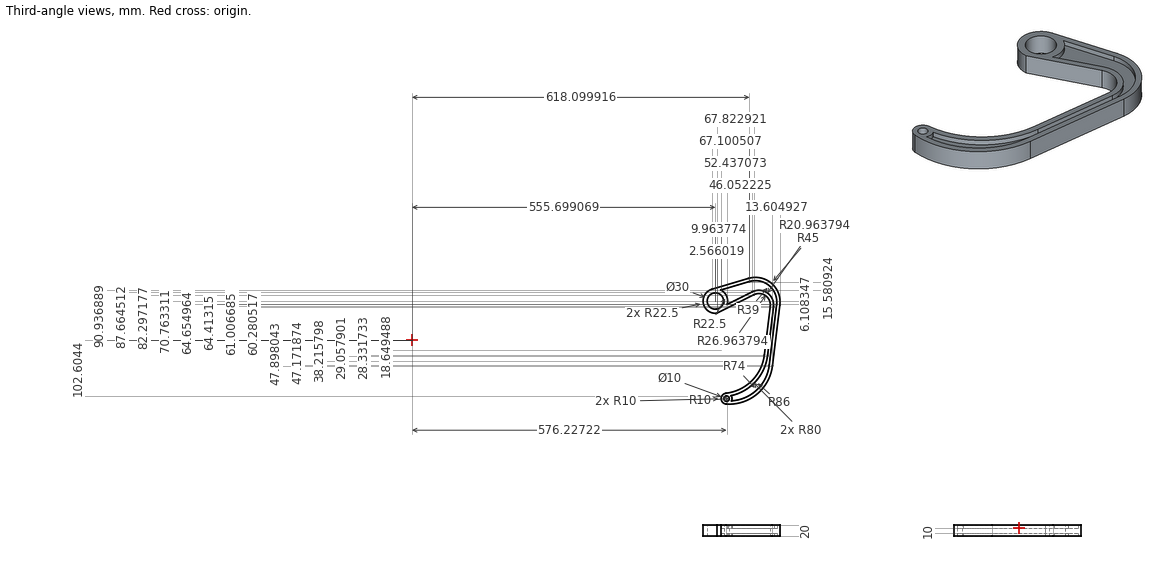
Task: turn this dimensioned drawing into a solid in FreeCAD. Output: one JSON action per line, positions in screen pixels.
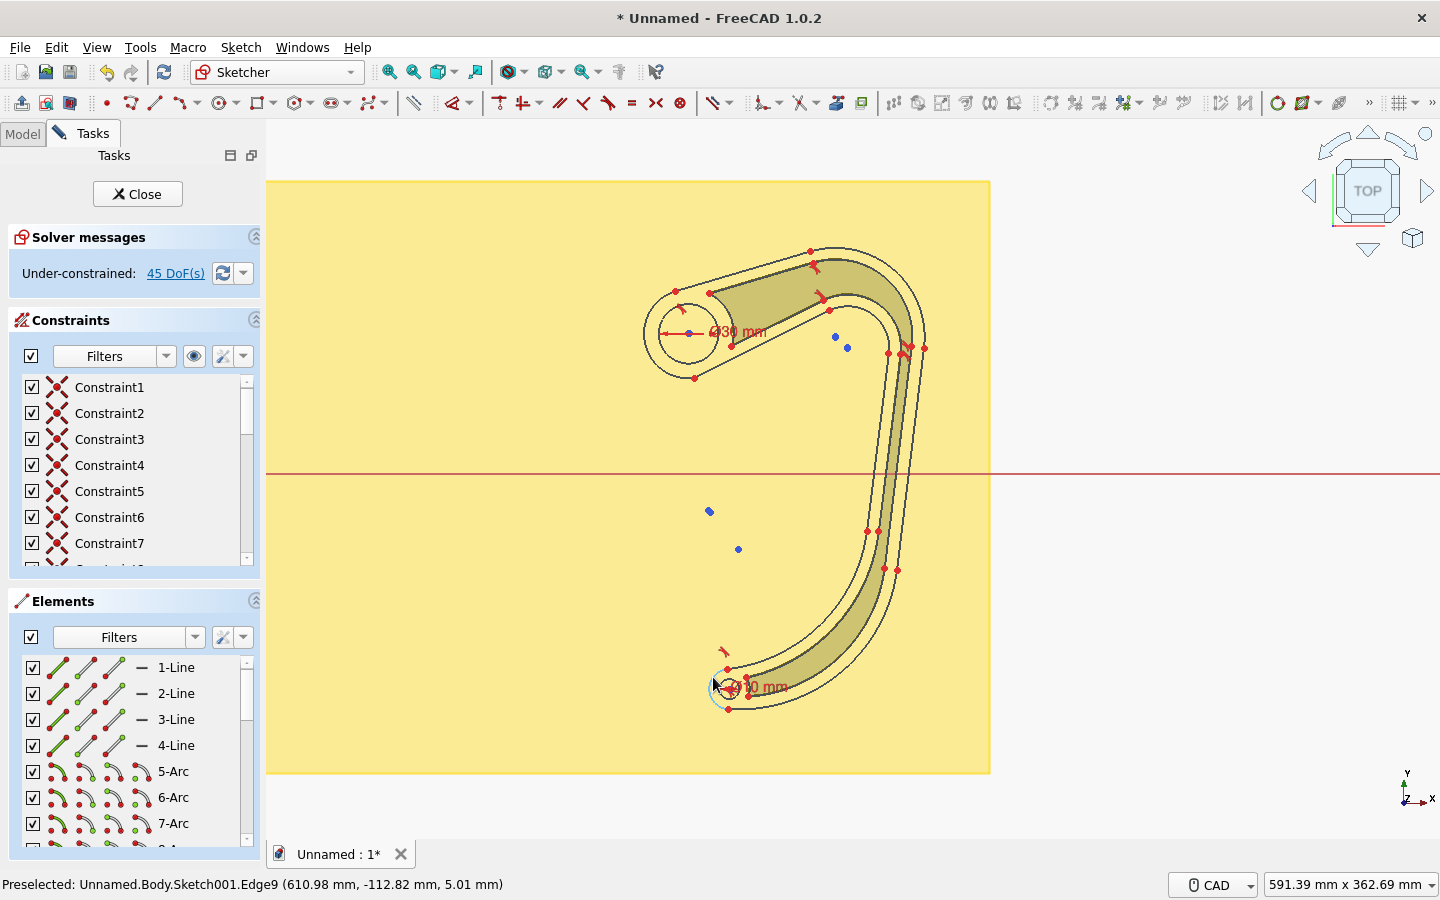
{"action": "left_click", "coordinate": [740, 285]}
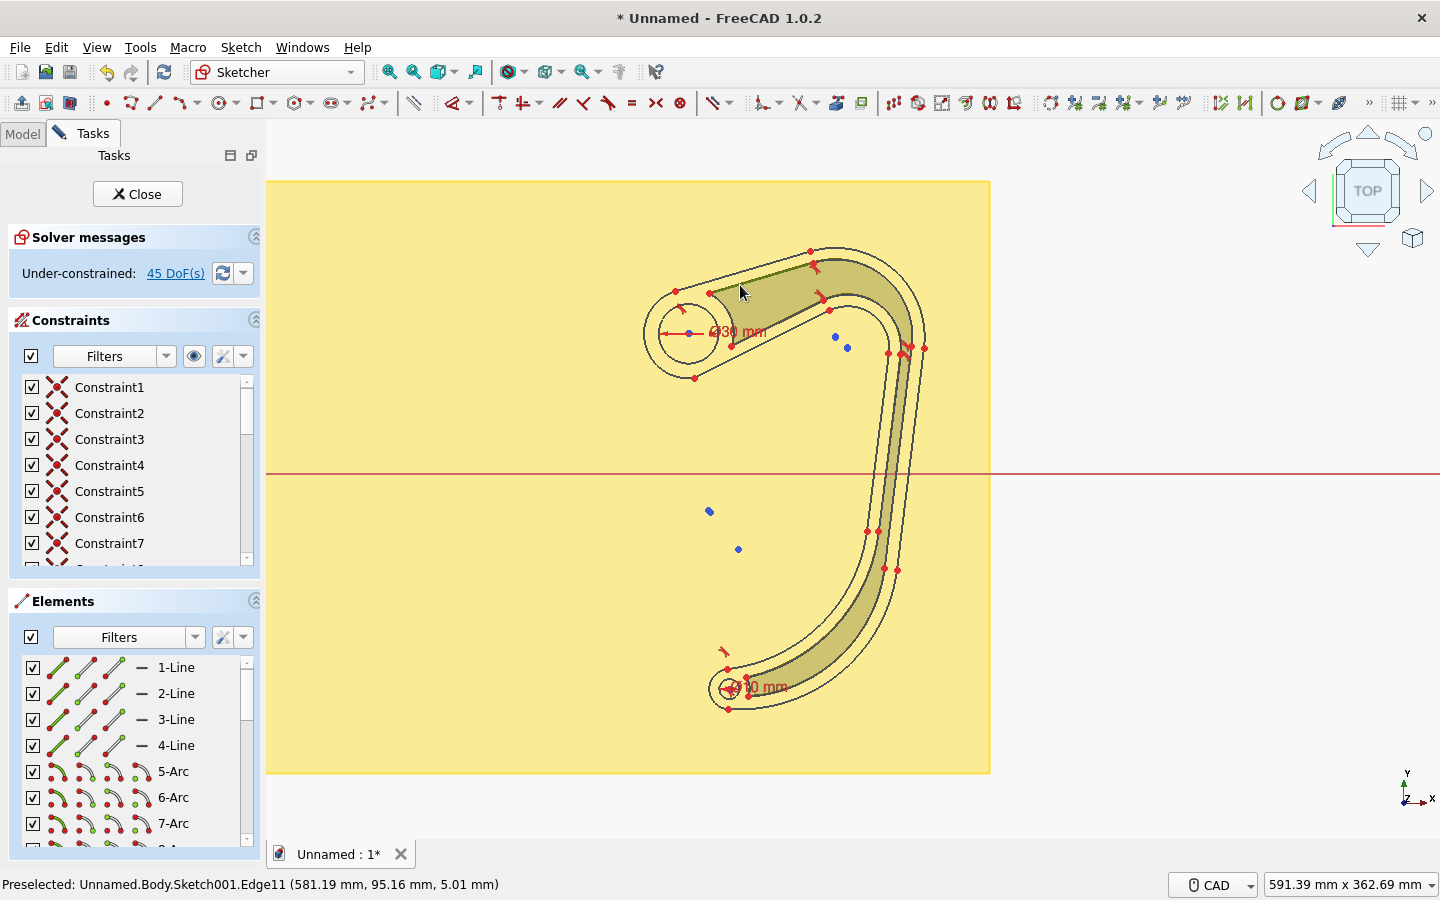
{"action": "left_click", "coordinate": [904, 302]}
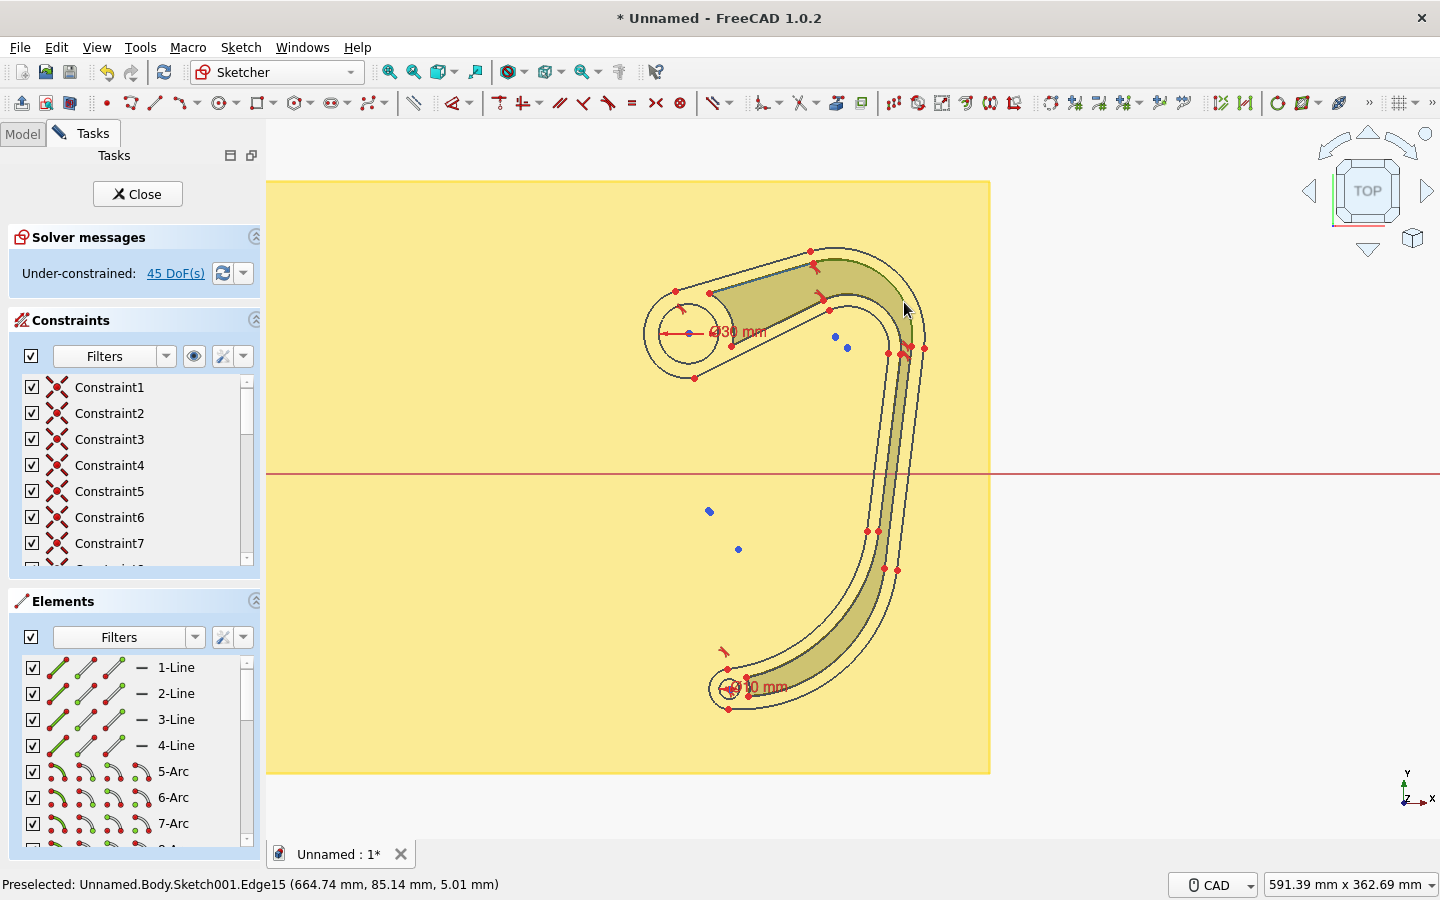
{"action": "left_click", "coordinate": [608, 104]}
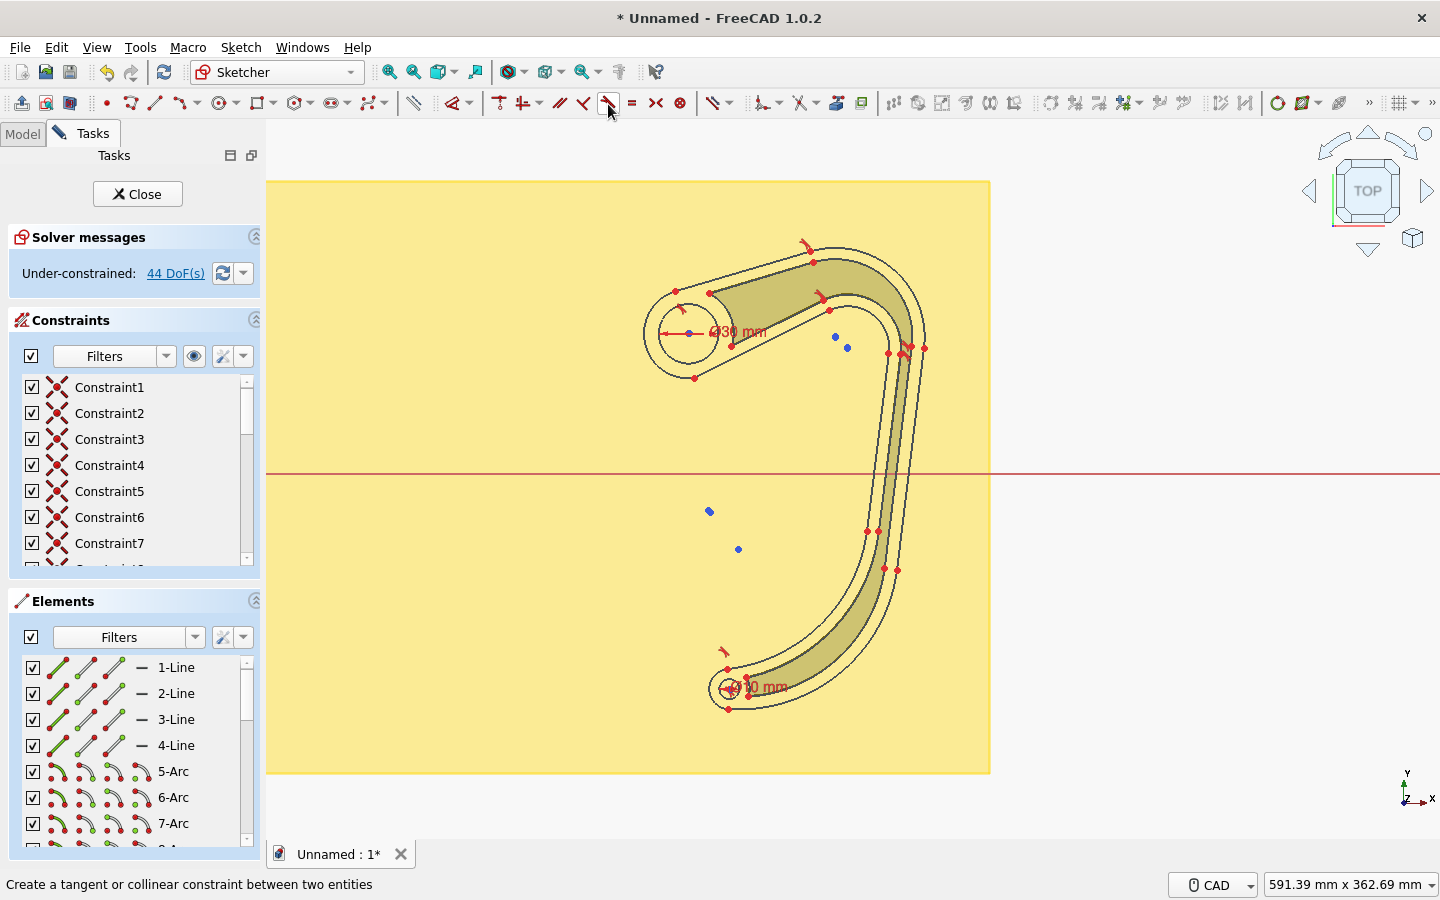
{"action": "scroll", "coordinate": [904, 413], "scroll_direction": "up", "scroll_amount": 2}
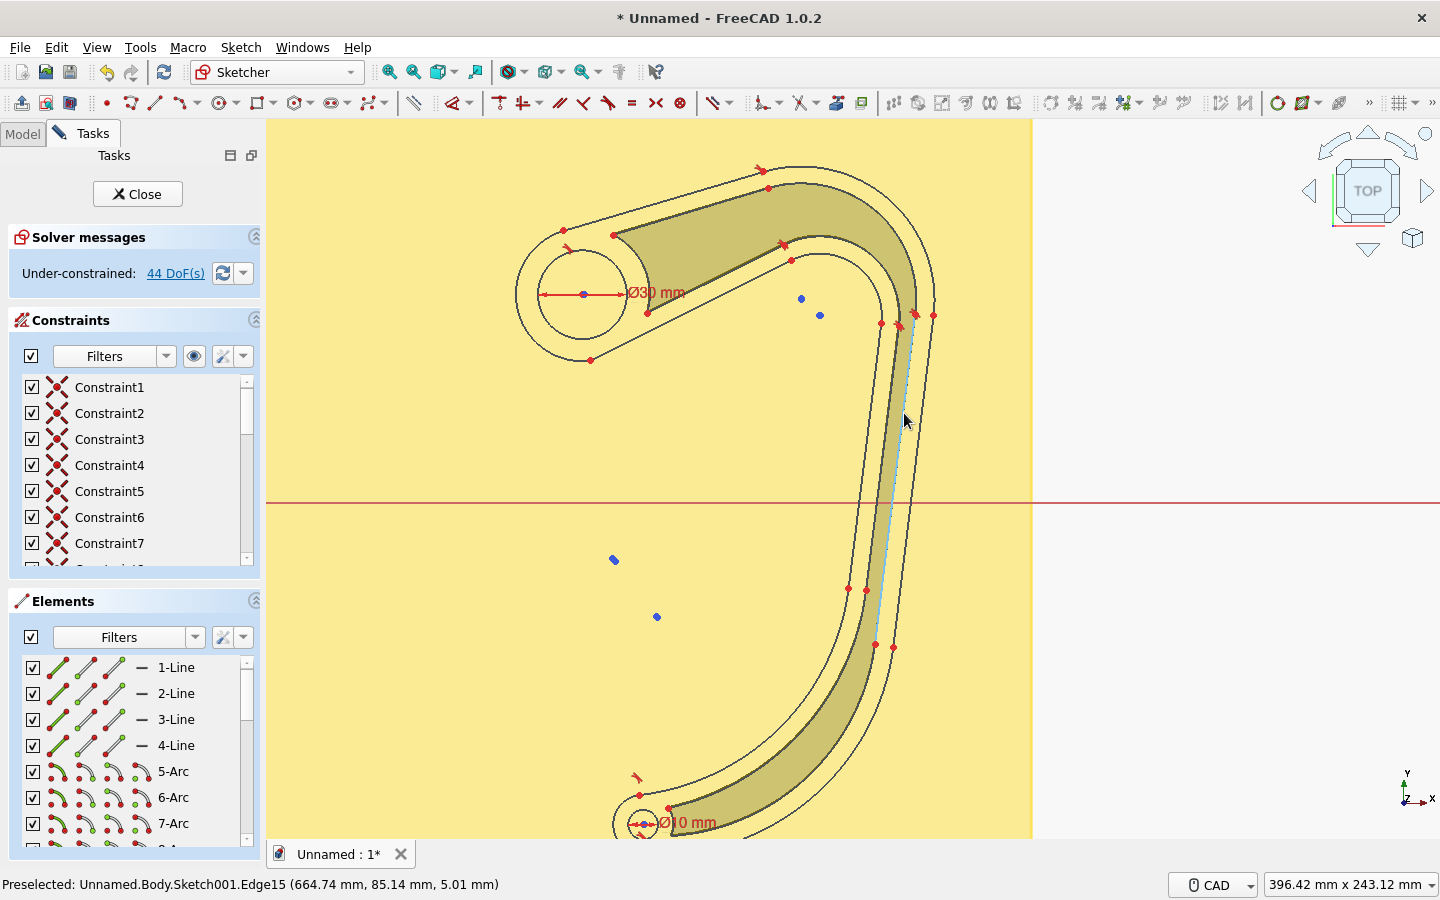
{"action": "left_click", "coordinate": [903, 413]}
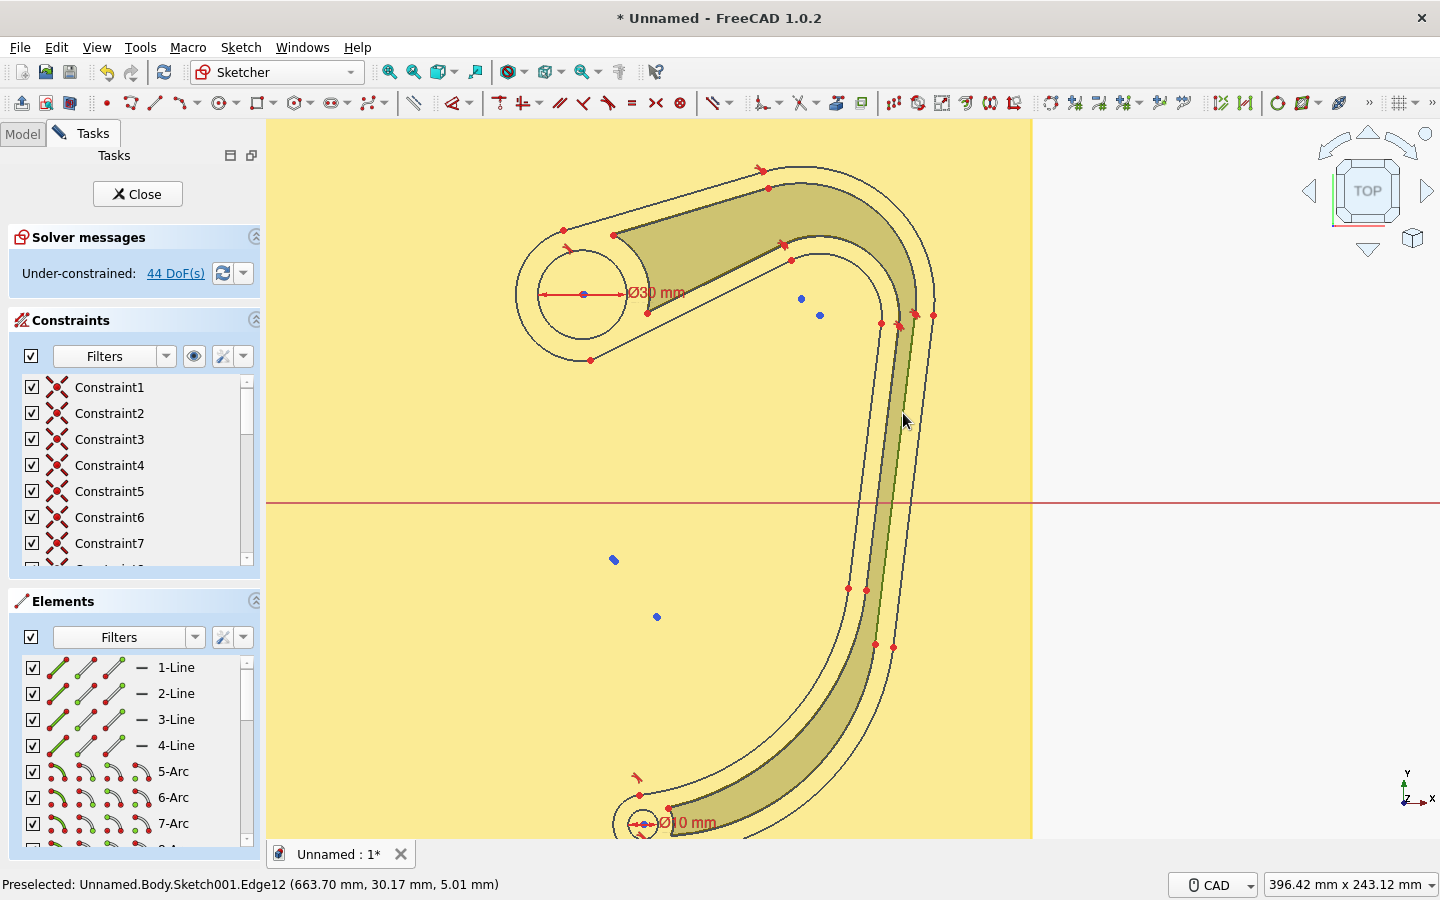
{"action": "left_click", "coordinate": [904, 247]}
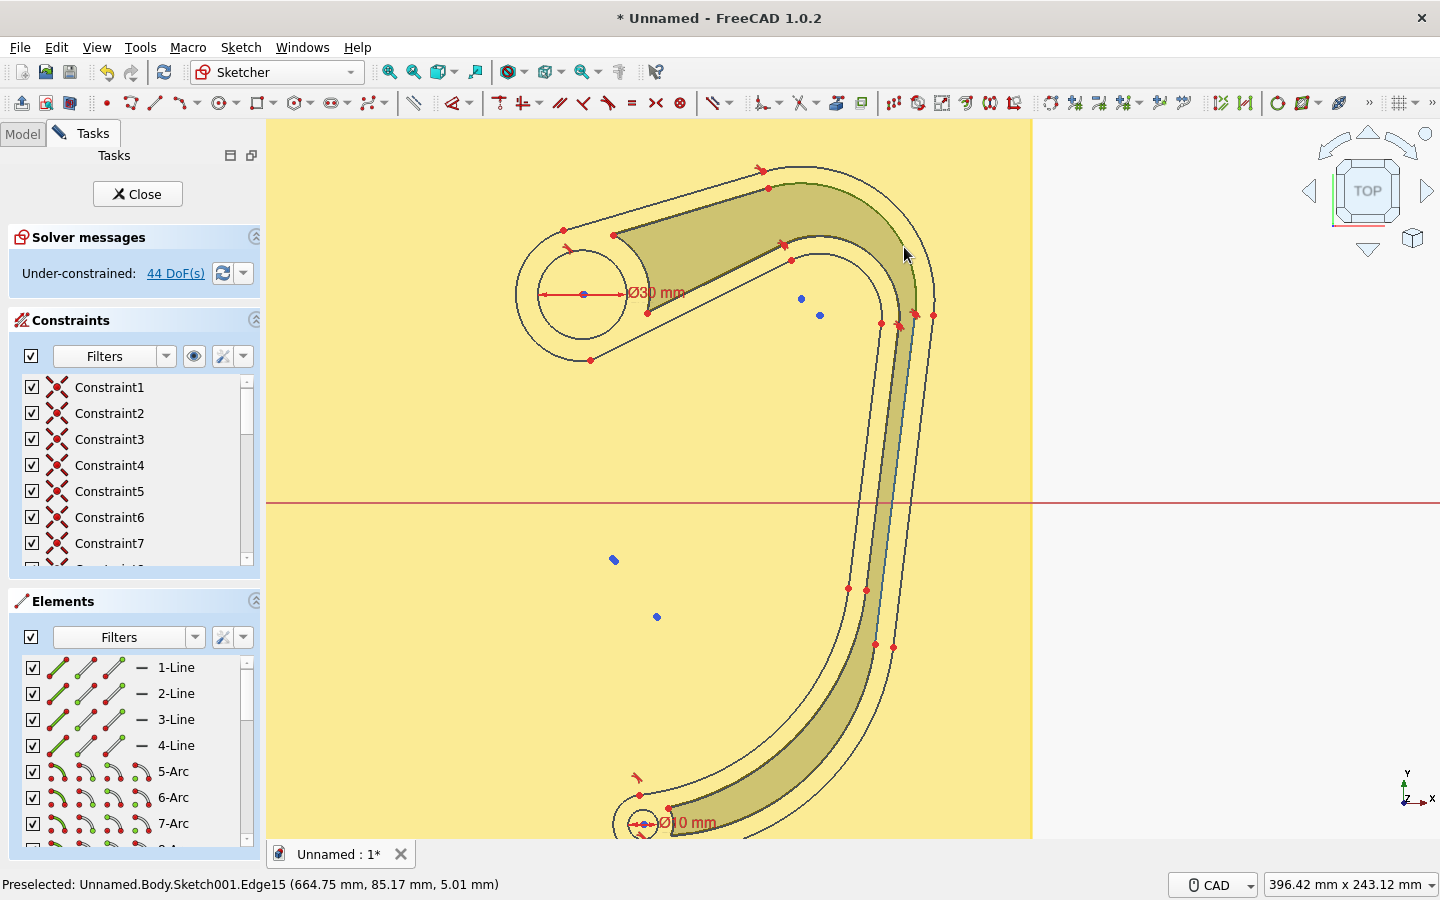
{"action": "left_click", "coordinate": [608, 104]}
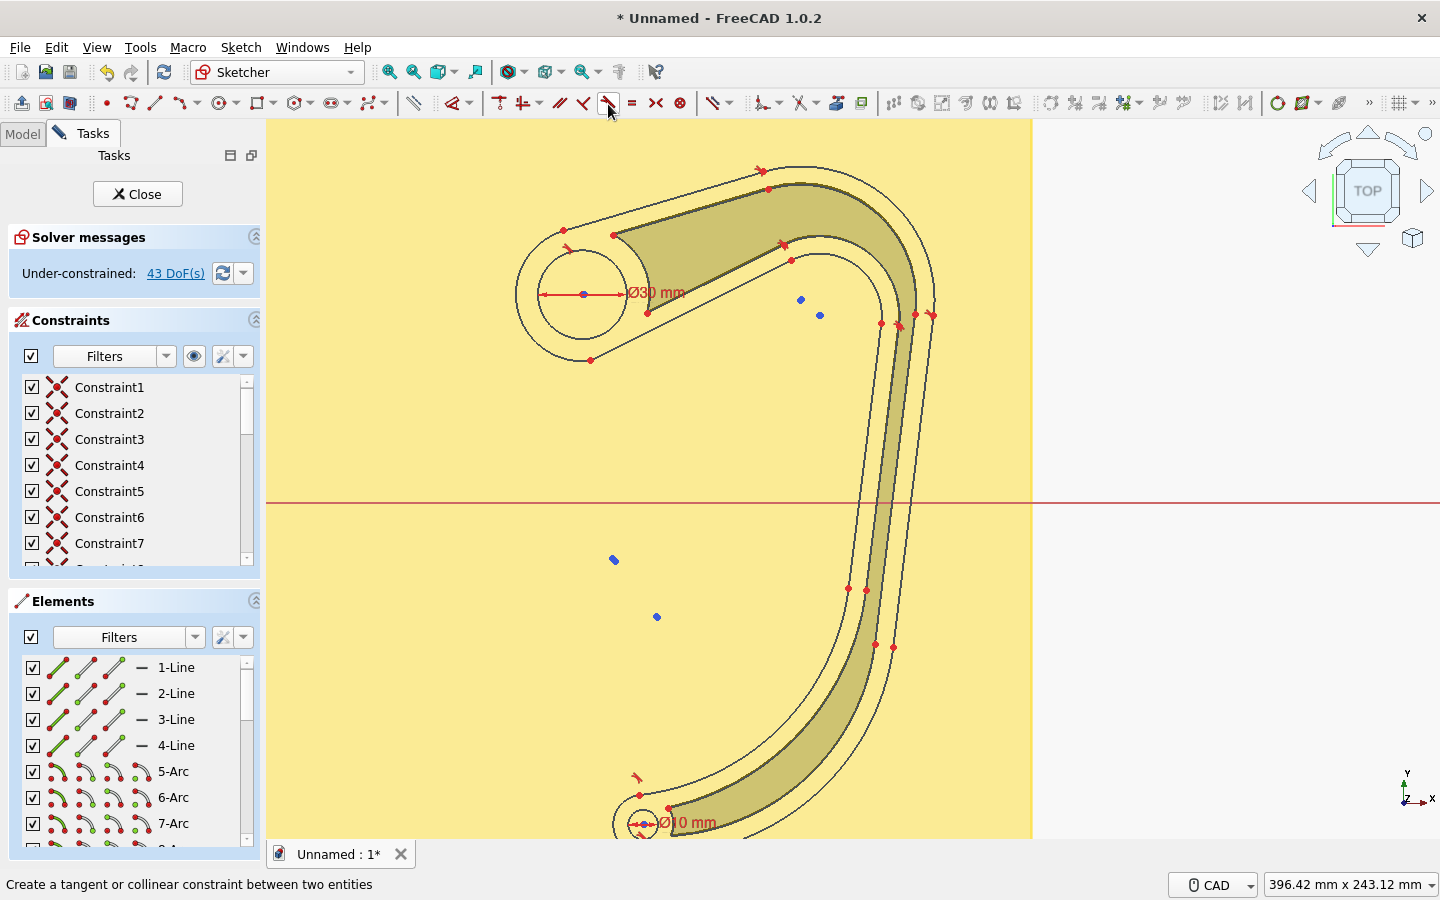
{"action": "left_click", "coordinate": [889, 405]}